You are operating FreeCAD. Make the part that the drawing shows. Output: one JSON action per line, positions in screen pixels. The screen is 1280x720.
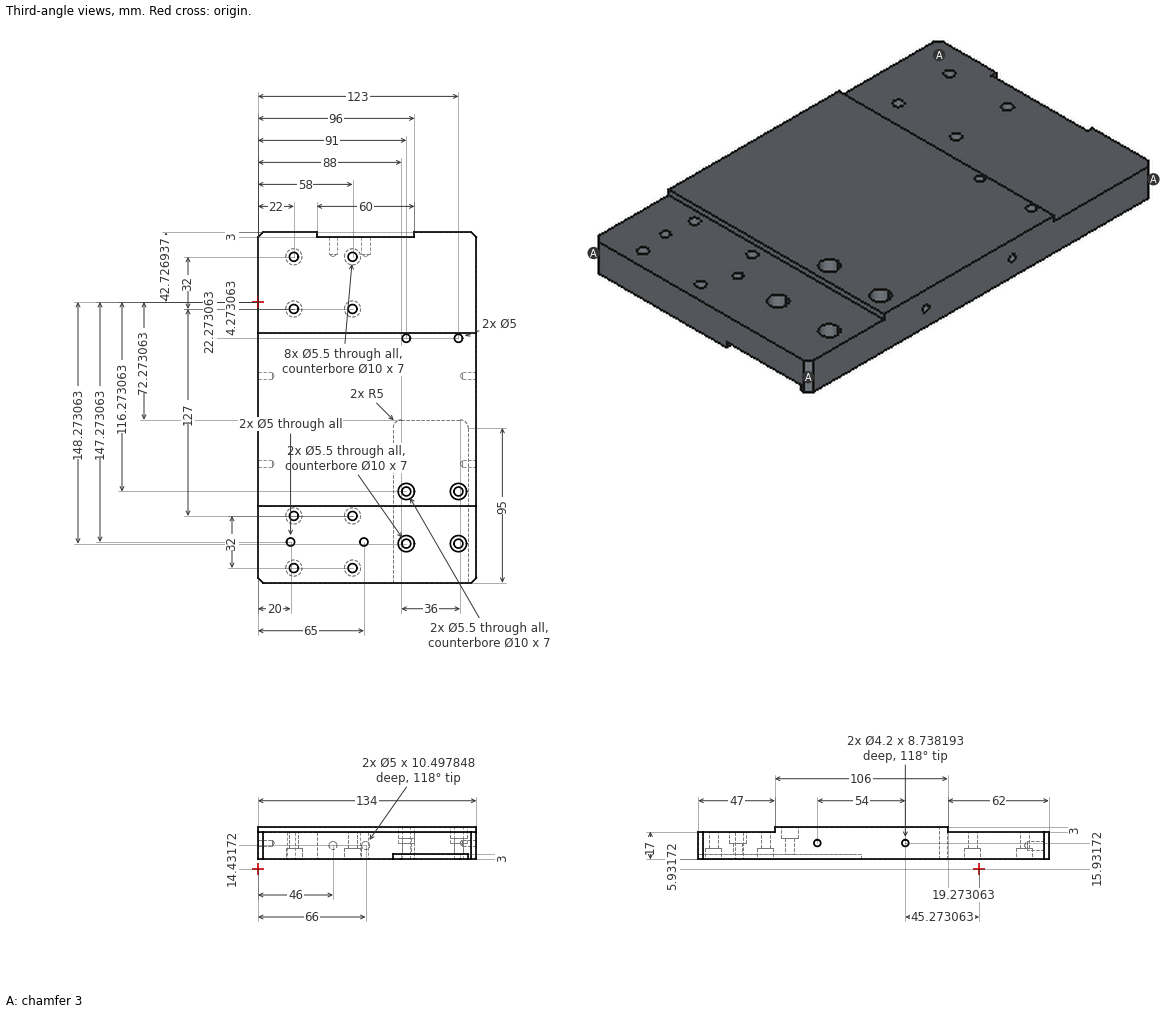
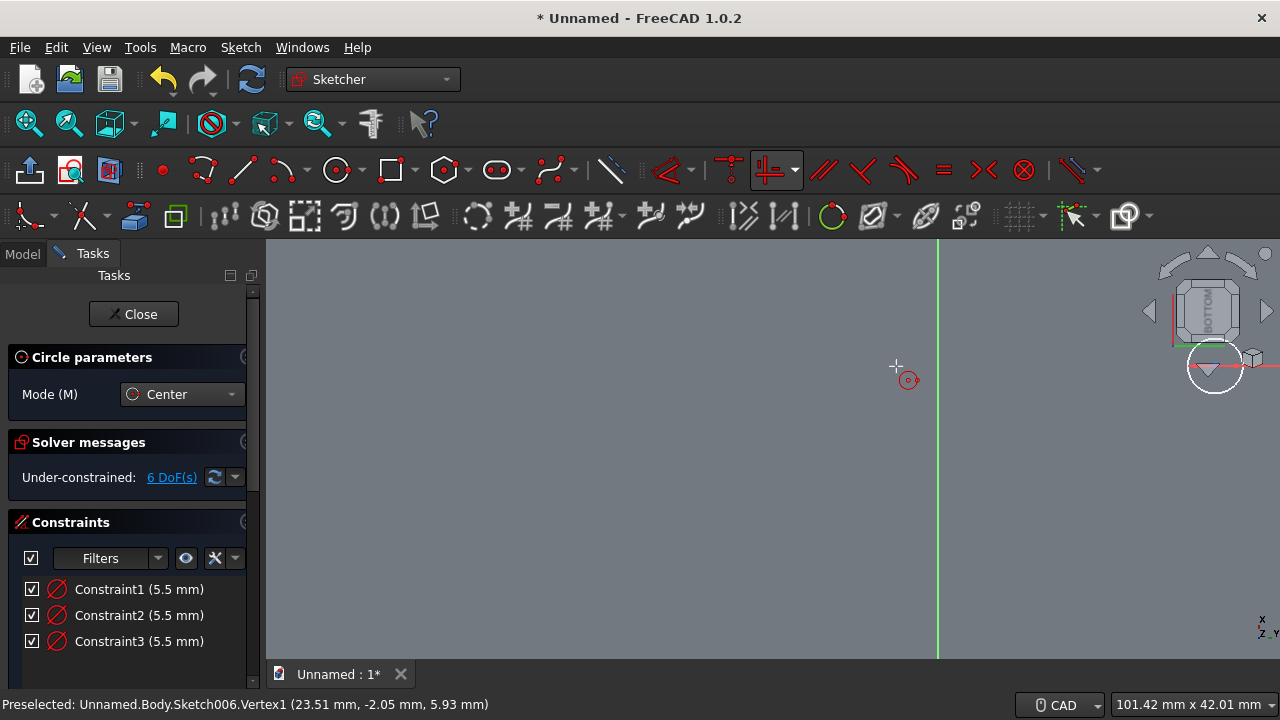
{"action": "left_click", "coordinate": [895, 365]}
{"action": "mouse_move", "coordinate": [915, 346]}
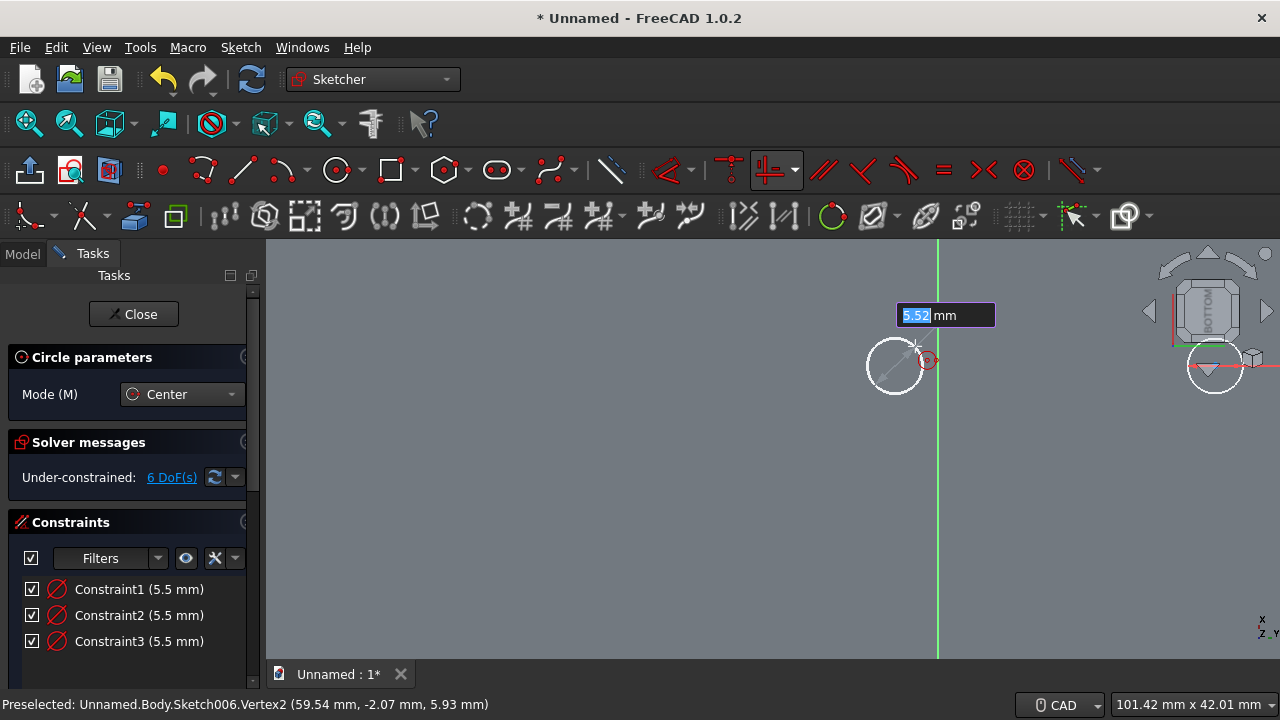
{"action": "type", "text": "5.5"}
{"action": "key", "text": "Return"}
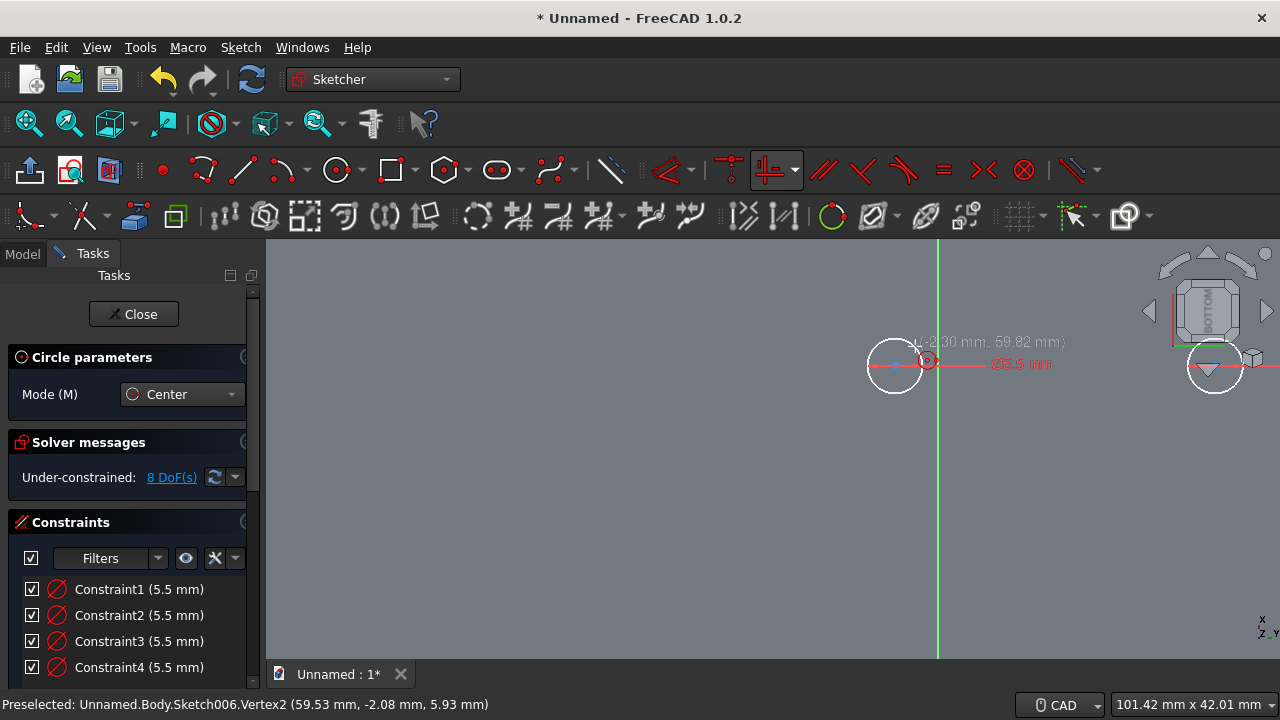
{"action": "scroll", "coordinate": [896, 366], "scroll_direction": "down", "scroll_amount": 6}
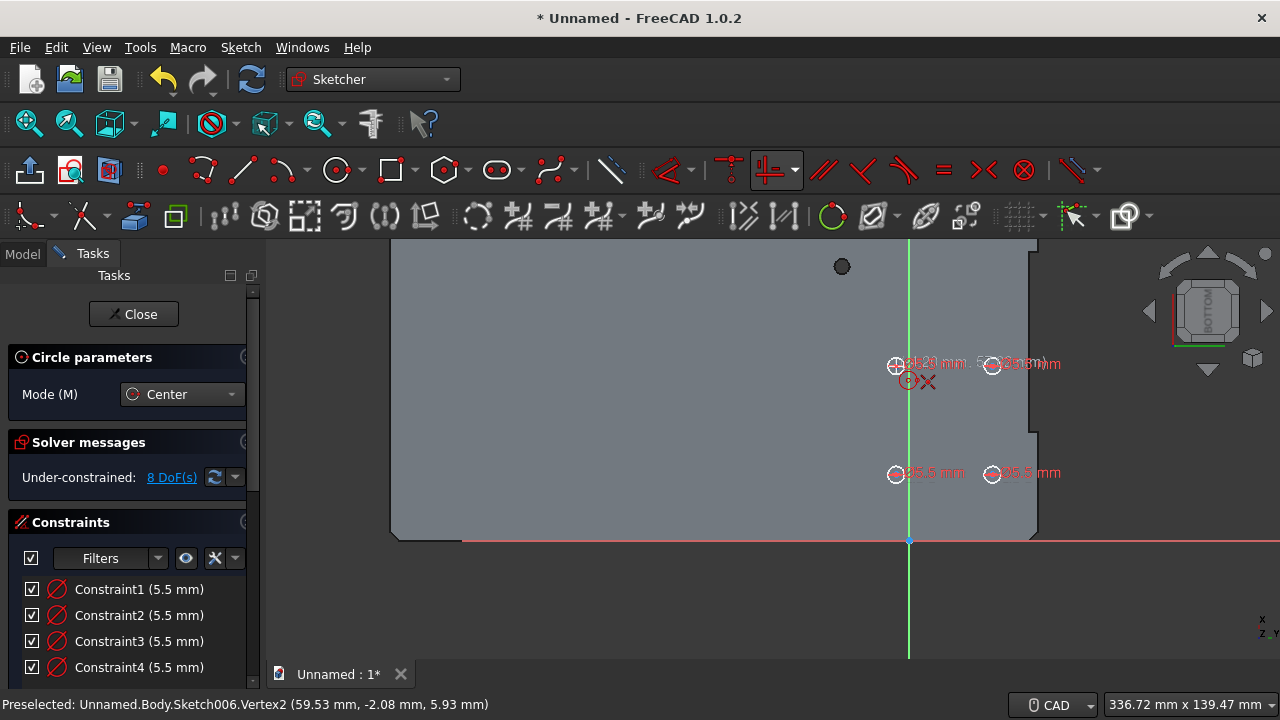
{"action": "scroll", "coordinate": [514, 366], "scroll_direction": "up", "scroll_amount": 6}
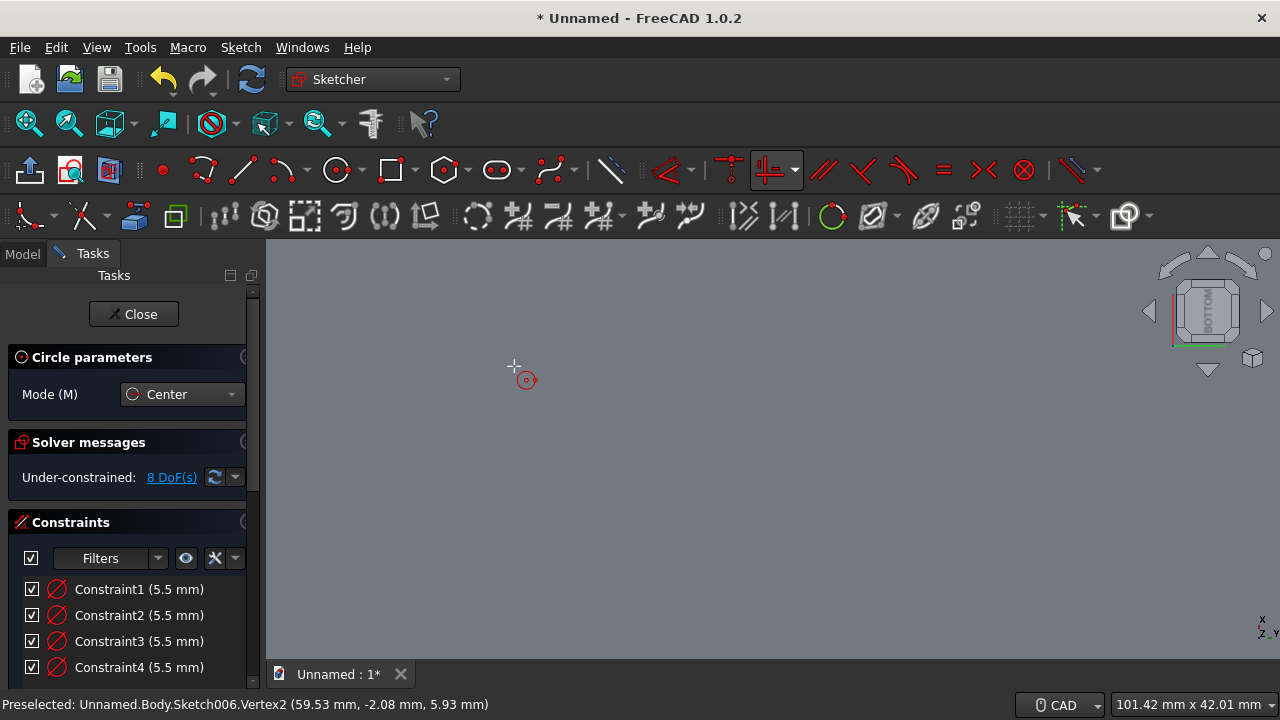
{"action": "left_click", "coordinate": [513, 365]}
{"action": "mouse_move", "coordinate": [532, 346]}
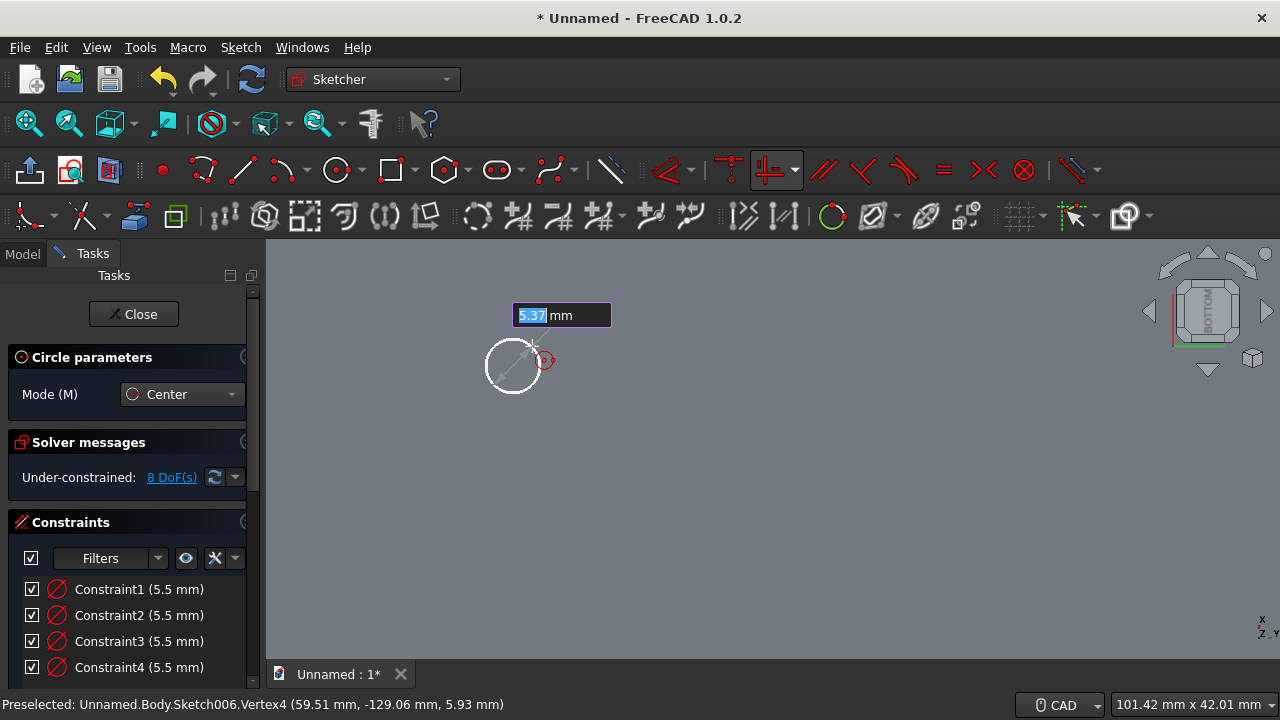
{"action": "type", "text": "5.5"}
{"action": "key", "text": "Return"}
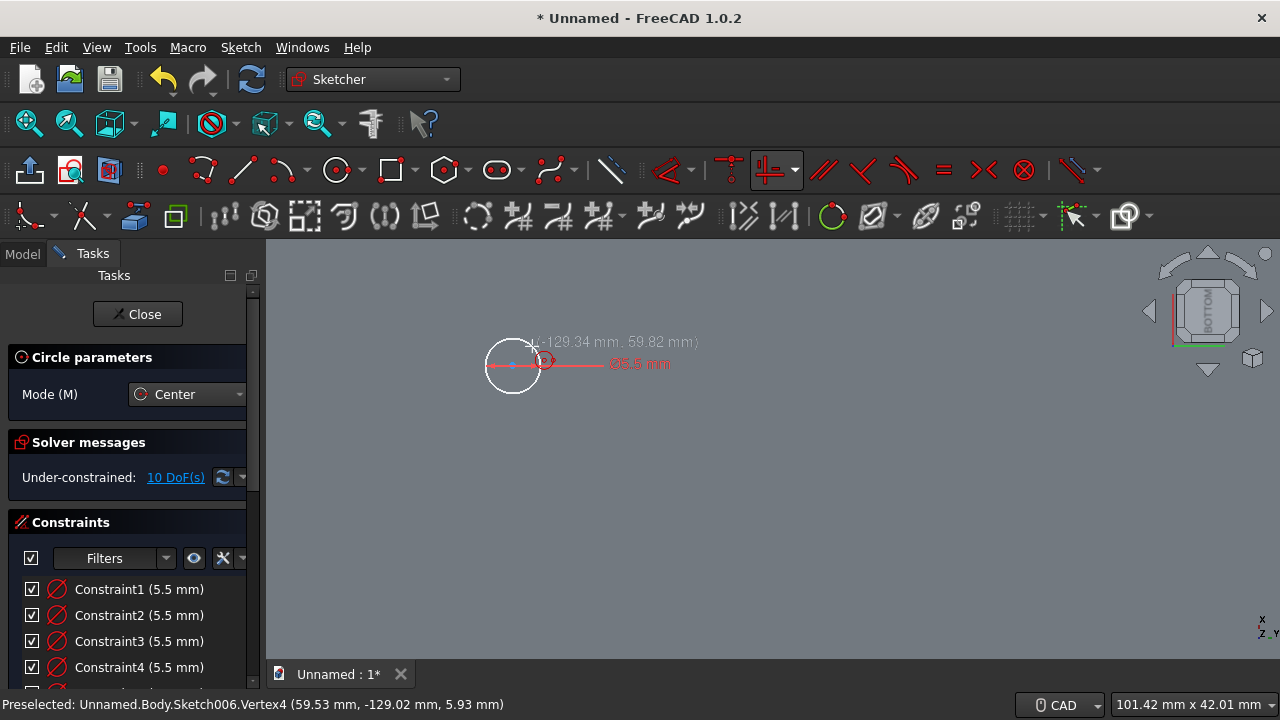
{"action": "scroll", "coordinate": [514, 366], "scroll_direction": "down", "scroll_amount": 6}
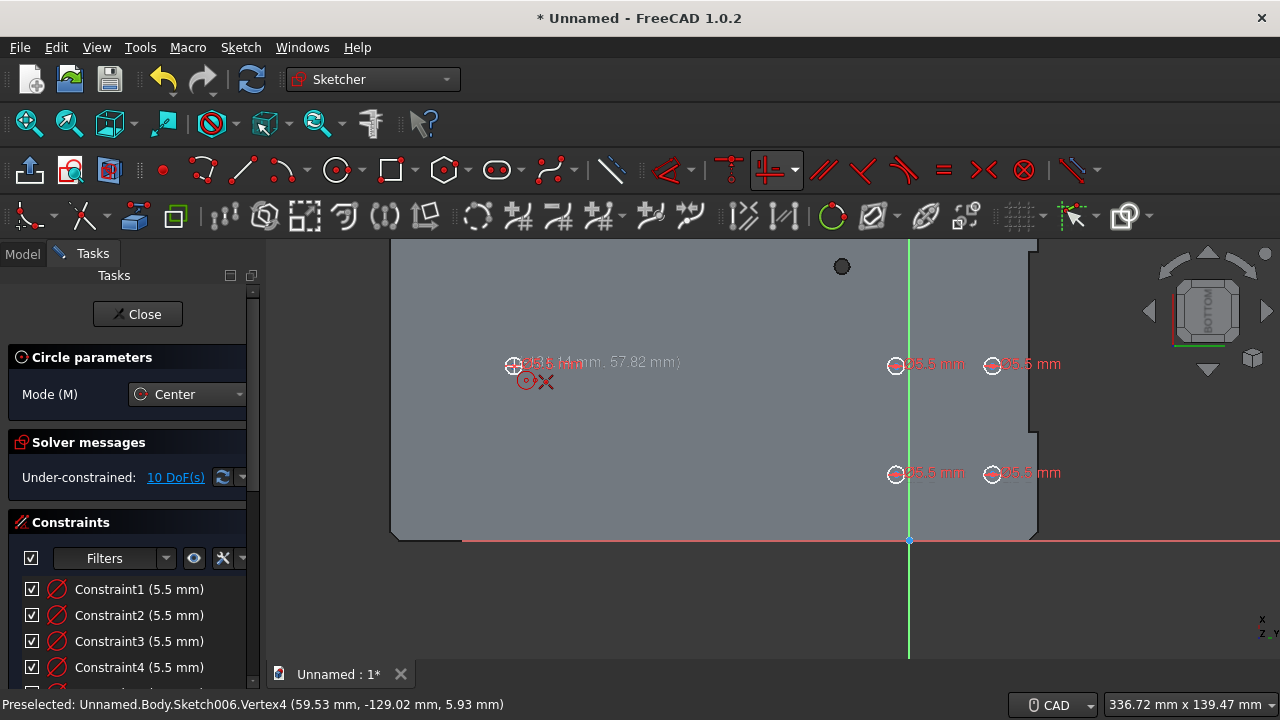
{"action": "scroll", "coordinate": [417, 366], "scroll_direction": "up", "scroll_amount": 6}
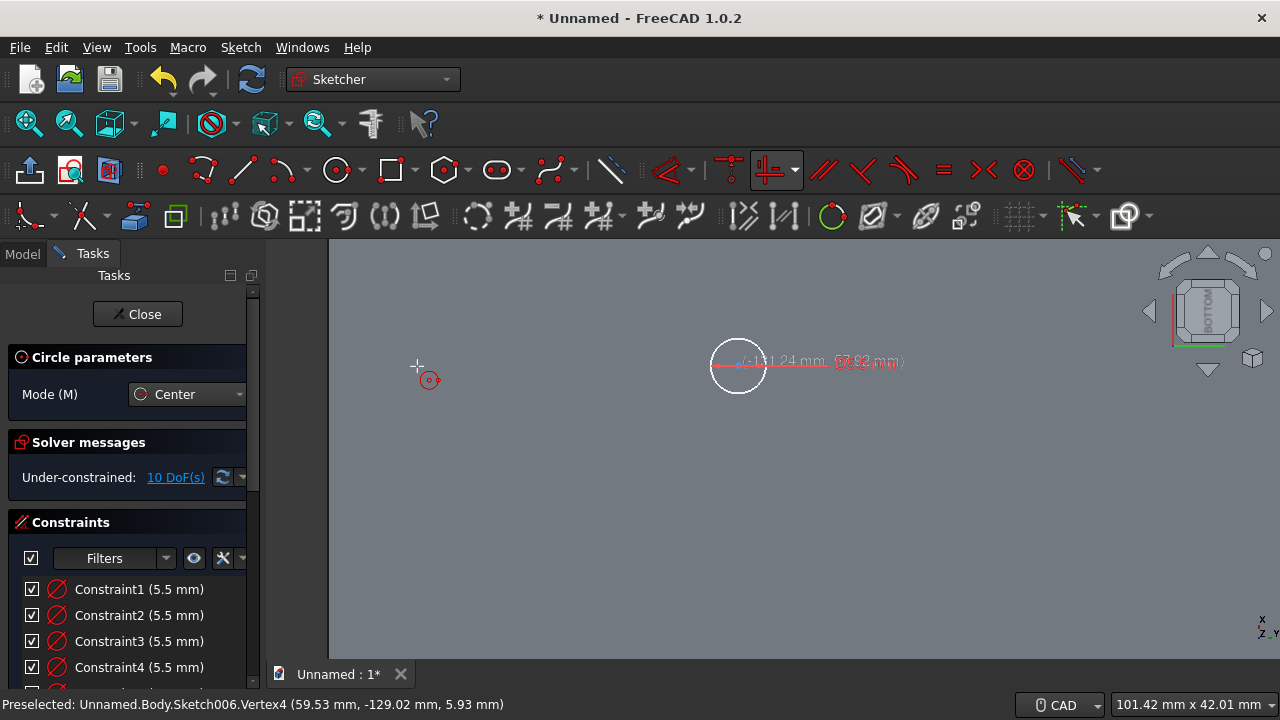
{"action": "left_click", "coordinate": [418, 365]}
{"action": "mouse_move", "coordinate": [437, 346]}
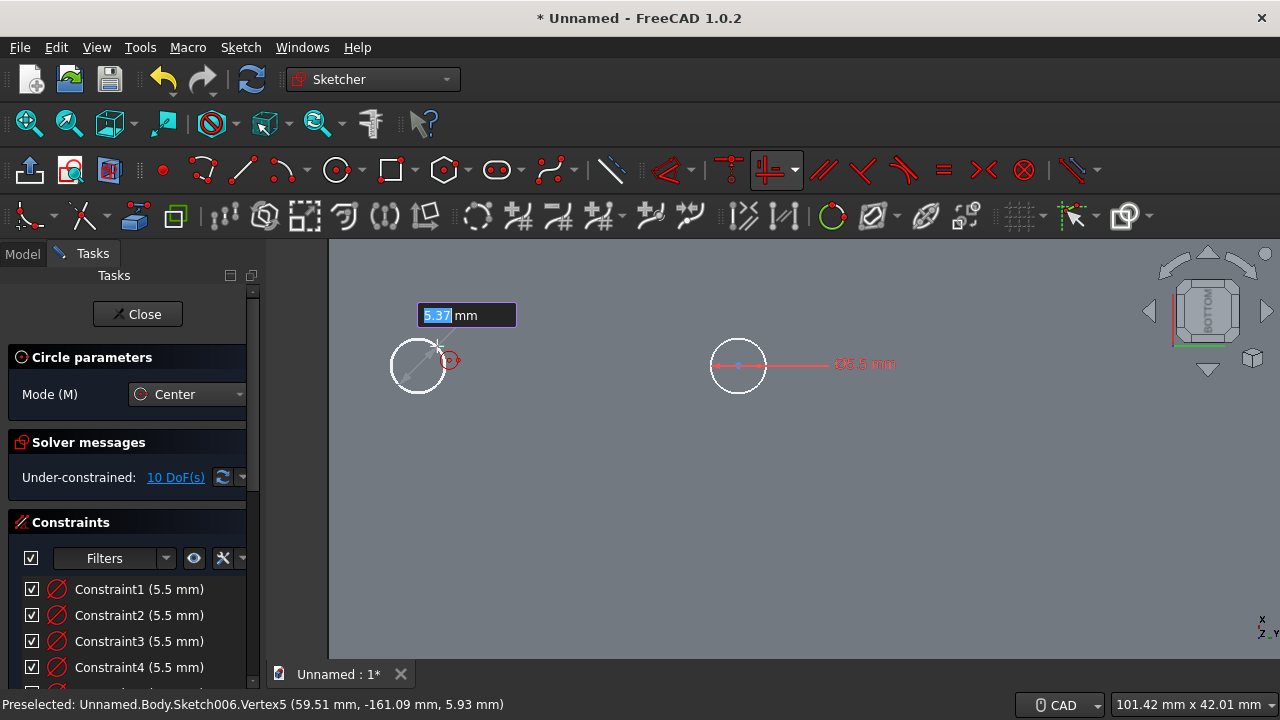
{"action": "type", "text": "5.5"}
{"action": "key", "text": "Return"}